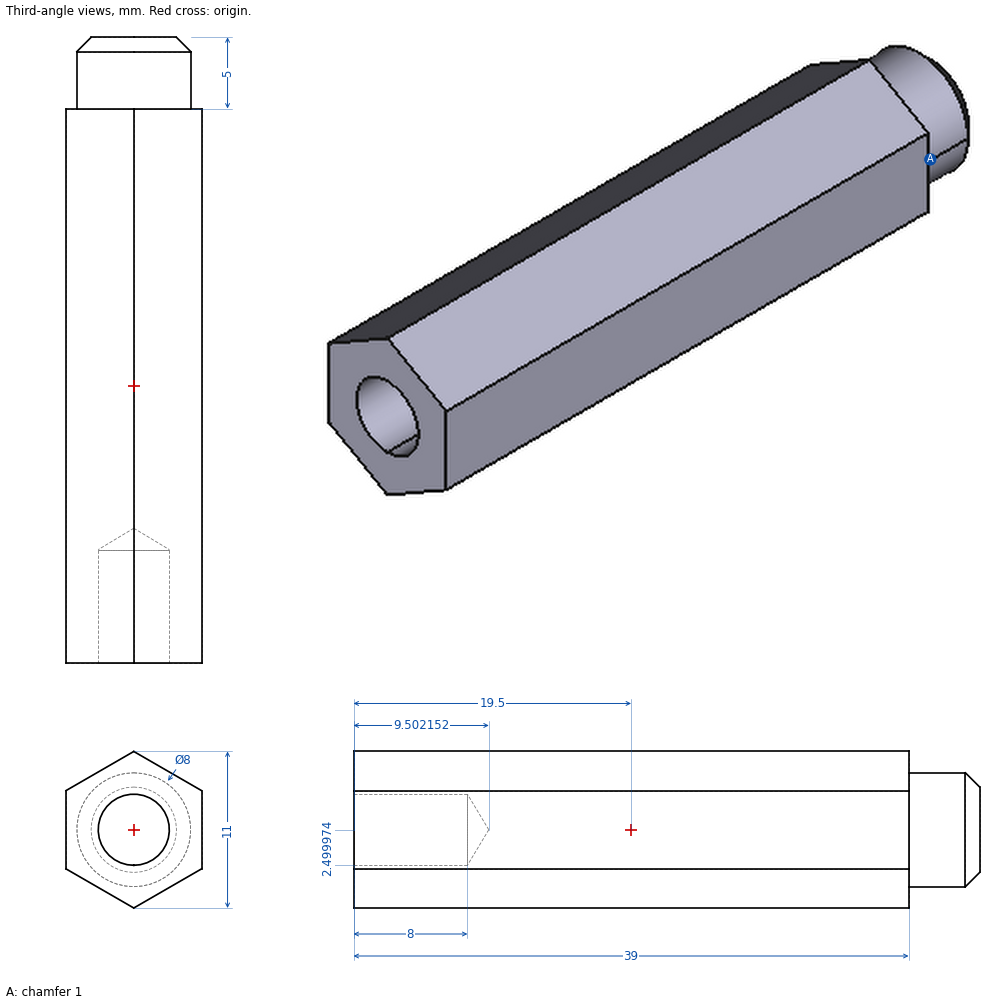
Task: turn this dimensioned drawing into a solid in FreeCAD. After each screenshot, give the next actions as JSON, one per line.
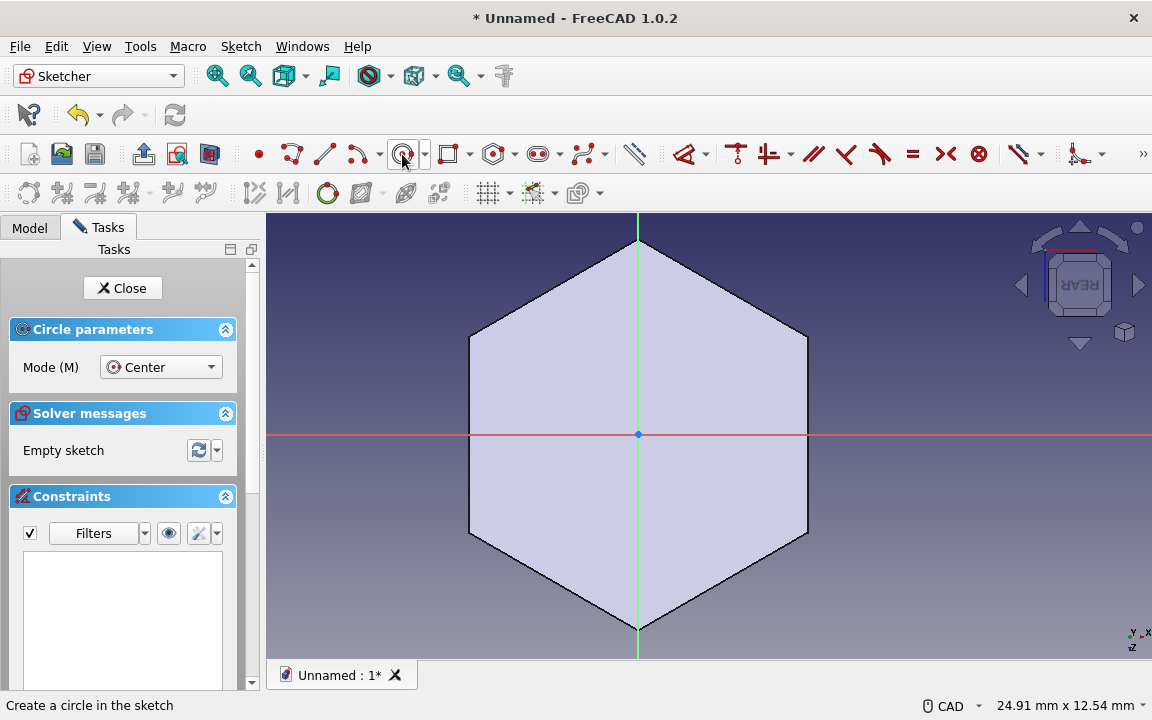
{"action": "left_click", "coordinate": [638, 435]}
{"action": "left_click", "coordinate": [739, 334]}
{"action": "key", "text": "Escape"}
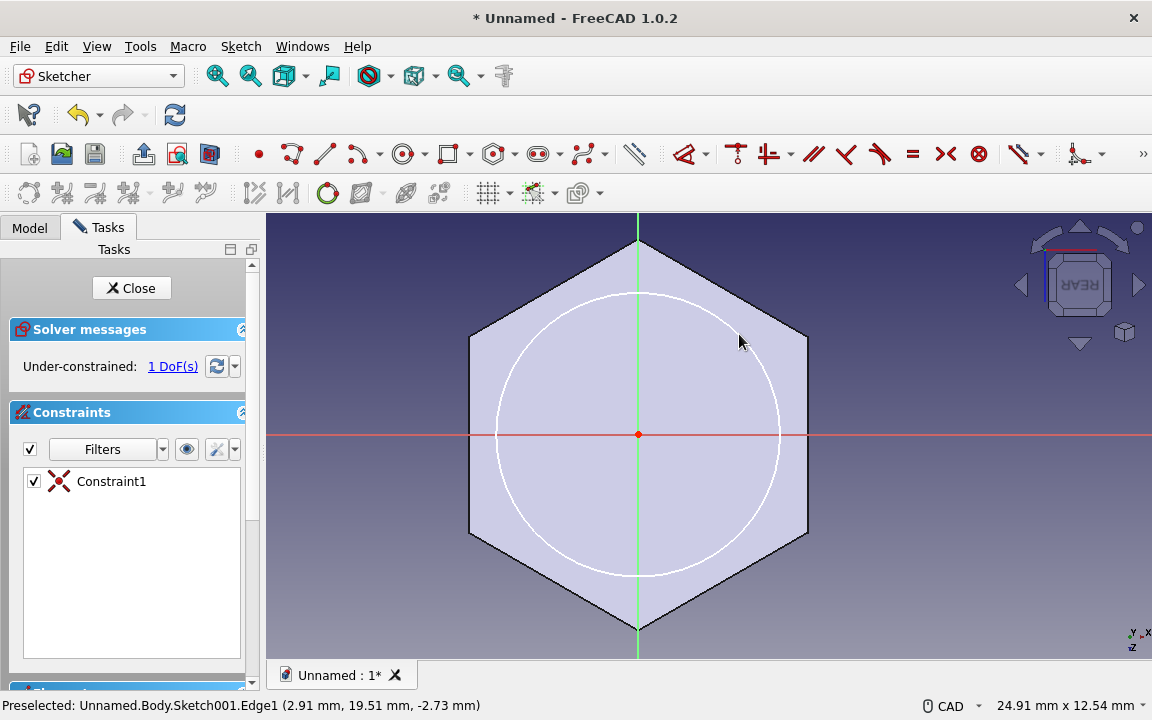
{"action": "key", "text": "d"}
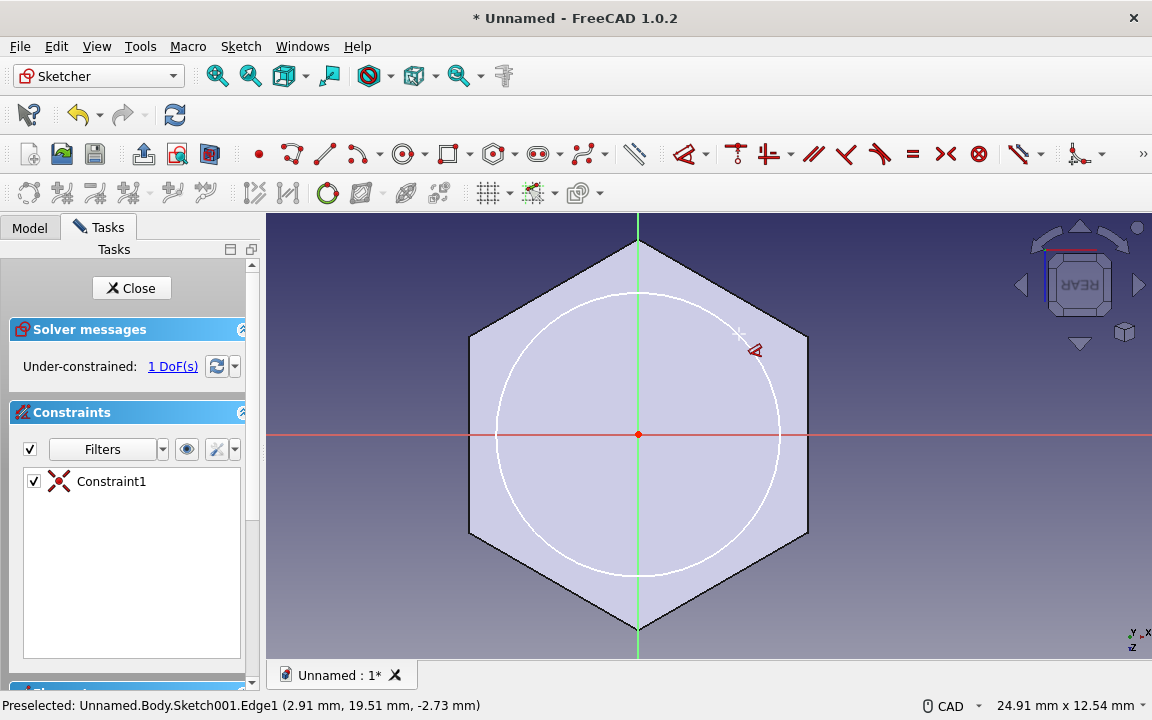
{"action": "left_click", "coordinate": [738, 334]}
{"action": "left_click", "coordinate": [761, 311]}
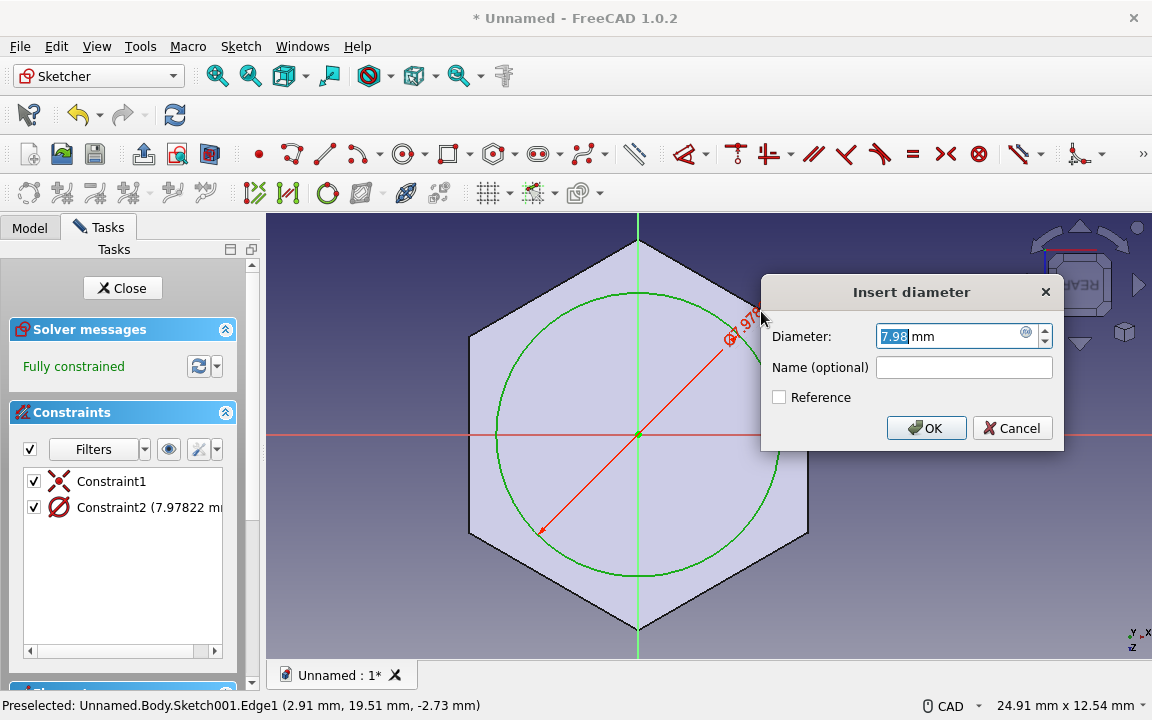
{"action": "type", "text": "8"}
{"action": "key", "text": "Return"}
{"action": "key", "text": "Escape"}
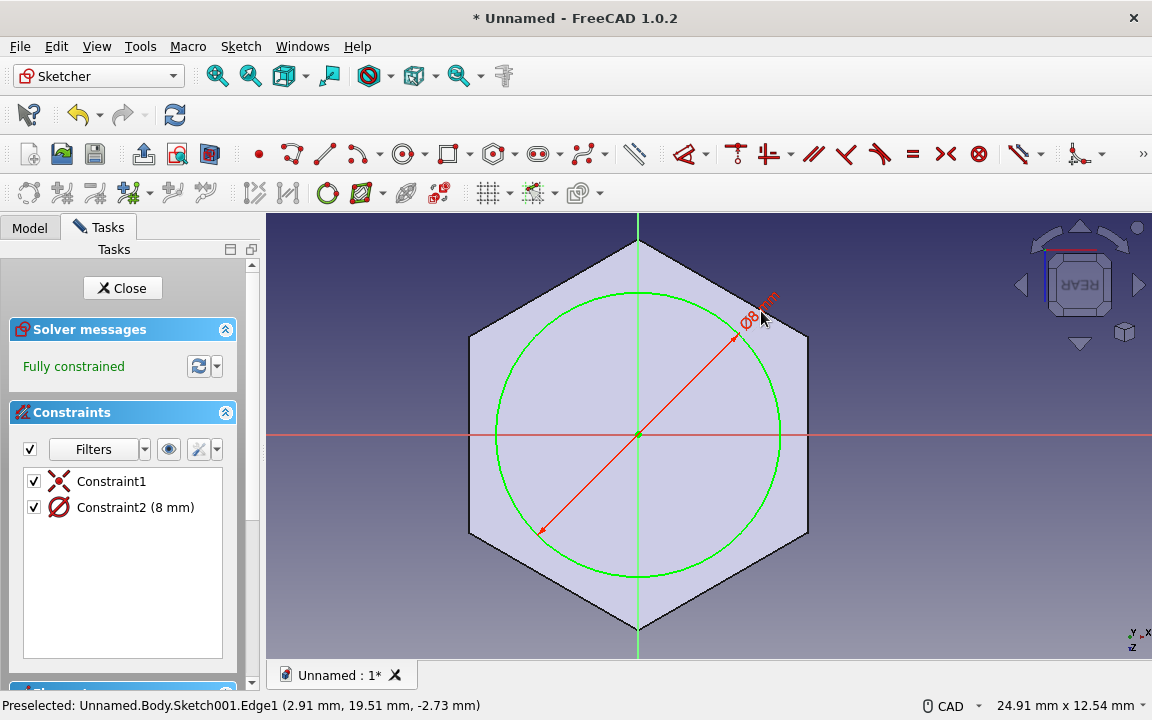
{"action": "left_click", "coordinate": [123, 288]}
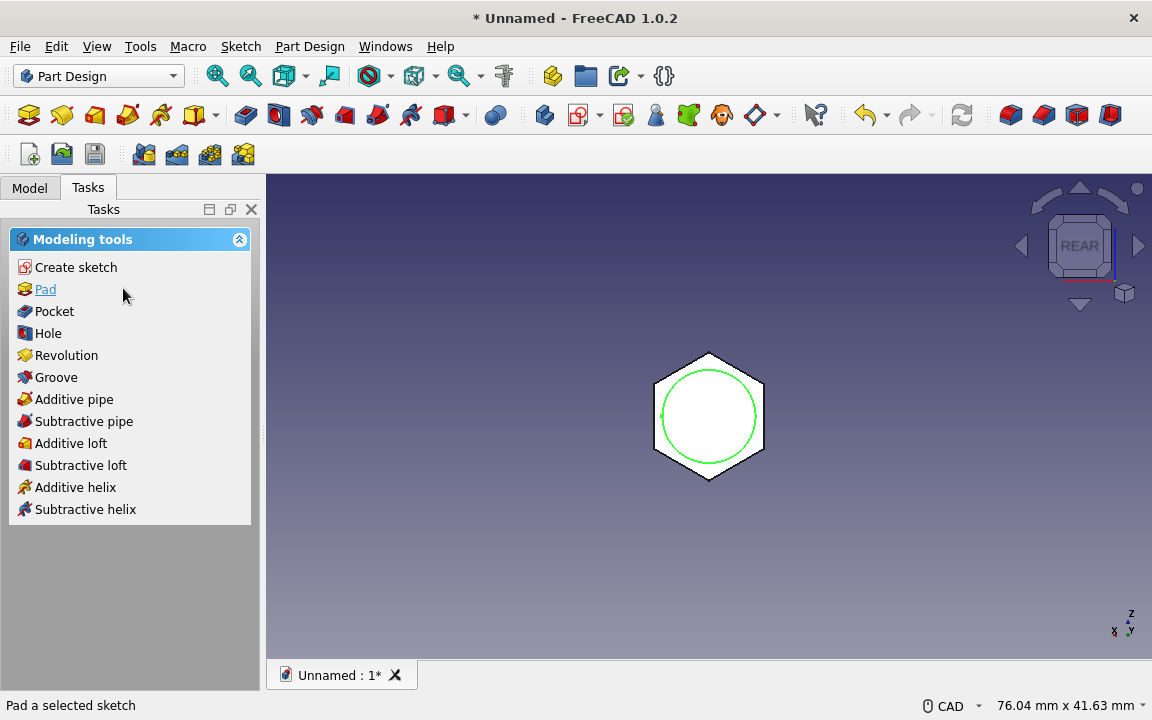
{"action": "left_click", "coordinate": [29, 116]}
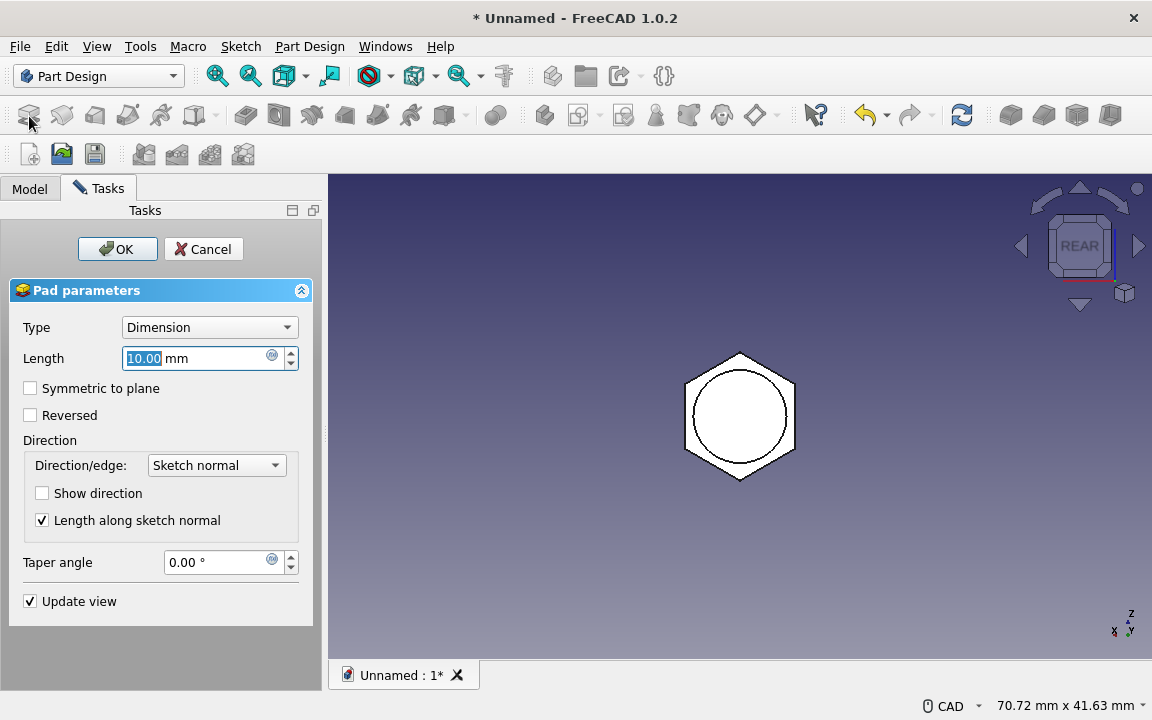
{"action": "type", "text": "5"}
{"action": "key", "text": "Tab"}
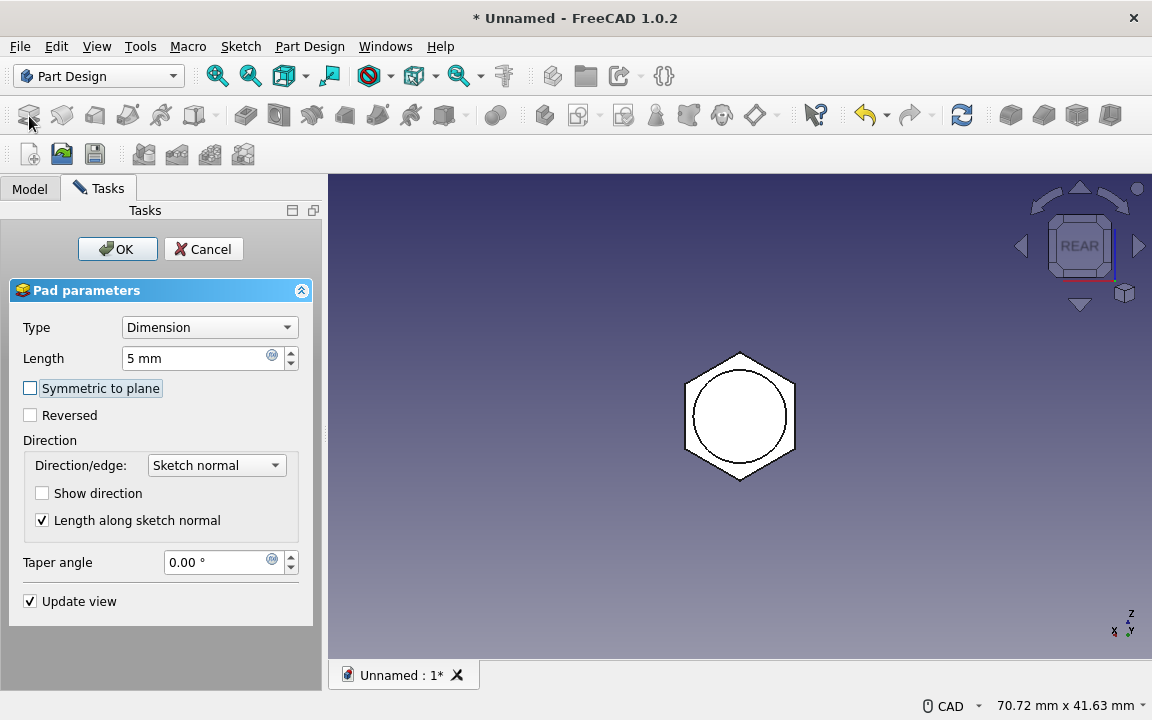
{"action": "left_click", "coordinate": [118, 249]}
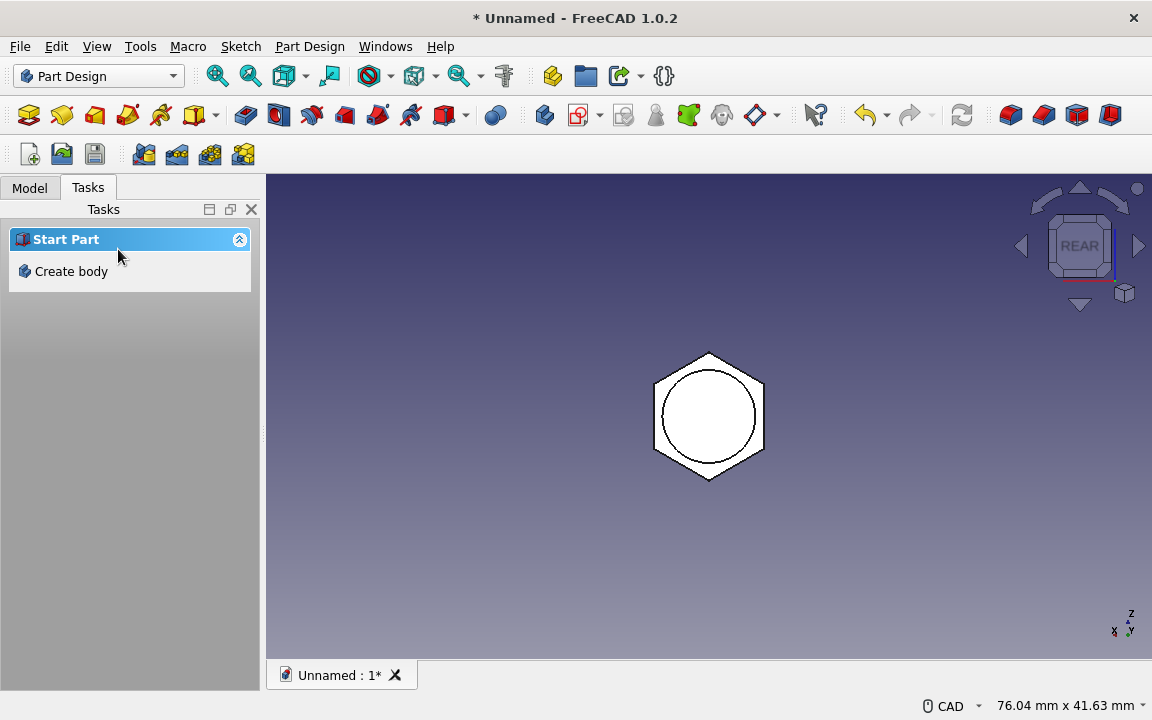
{"action": "left_click", "coordinate": [218, 76]}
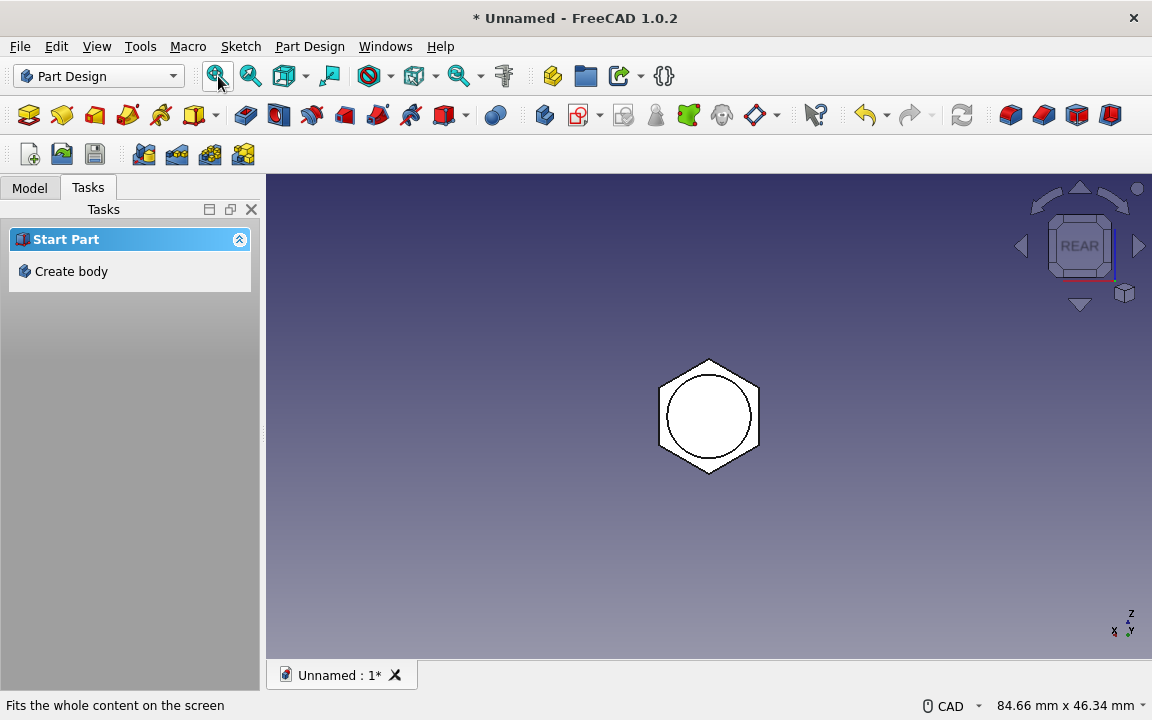
{"action": "left_click", "coordinate": [751, 415]}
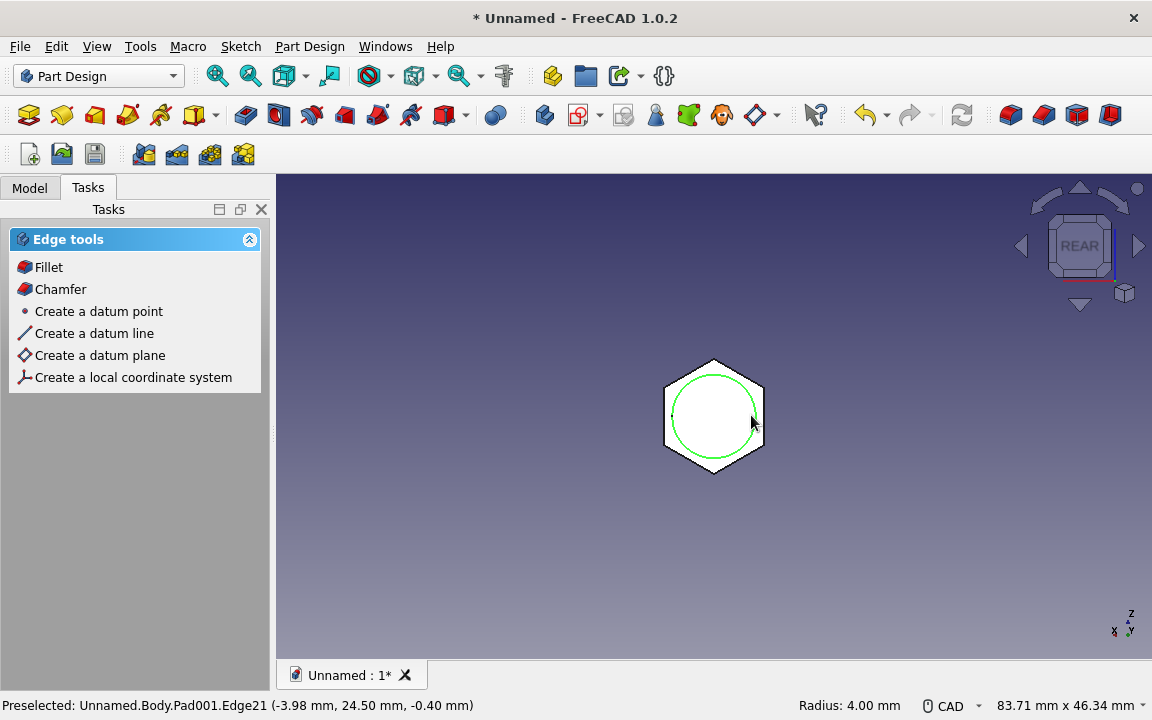
{"action": "left_click", "coordinate": [1044, 116]}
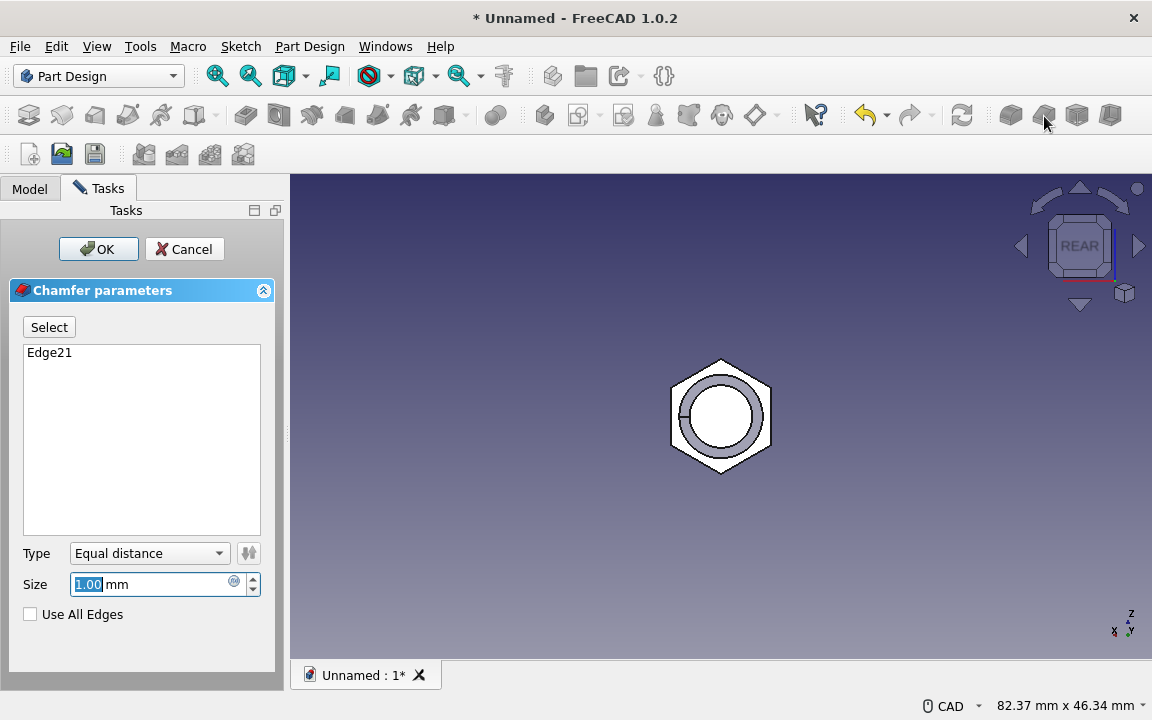
{"action": "type", "text": "1"}
{"action": "key", "text": "Tab"}